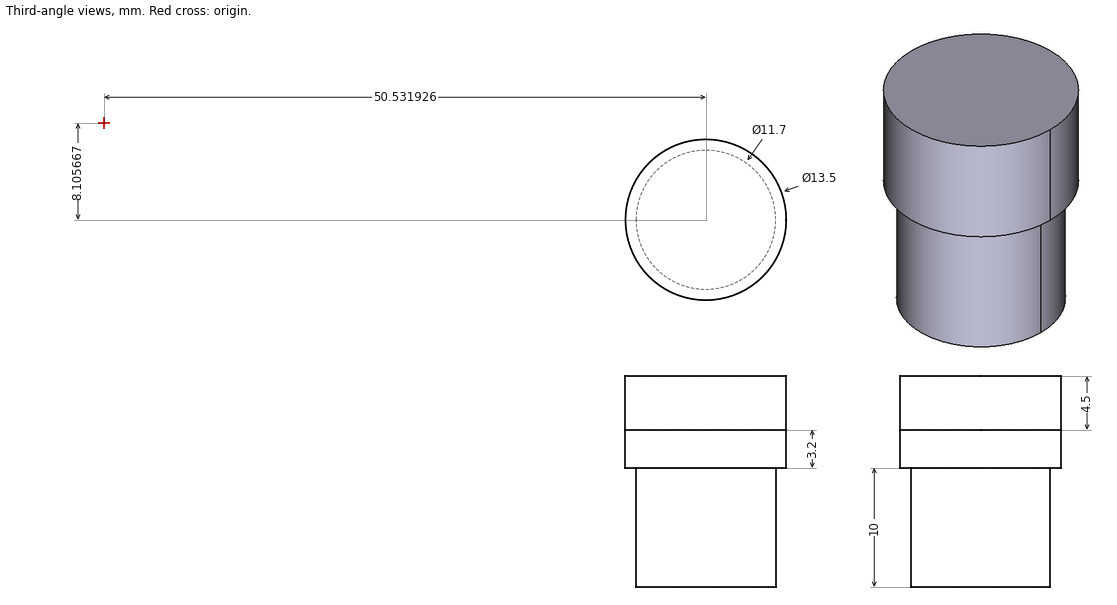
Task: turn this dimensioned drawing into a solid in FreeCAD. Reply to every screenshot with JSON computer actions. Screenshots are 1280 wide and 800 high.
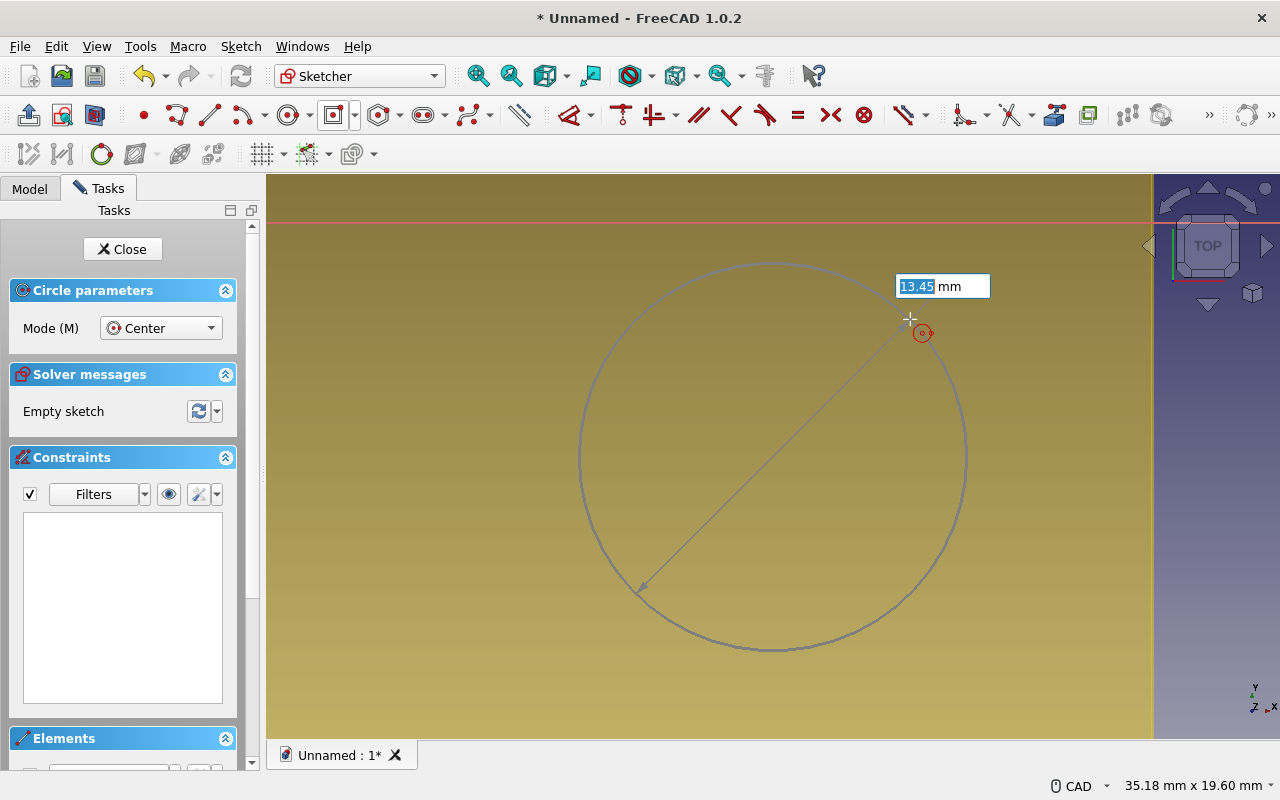
{"action": "type", "text": "13.5"}
{"action": "key", "text": "Return"}
{"action": "key", "text": "Escape"}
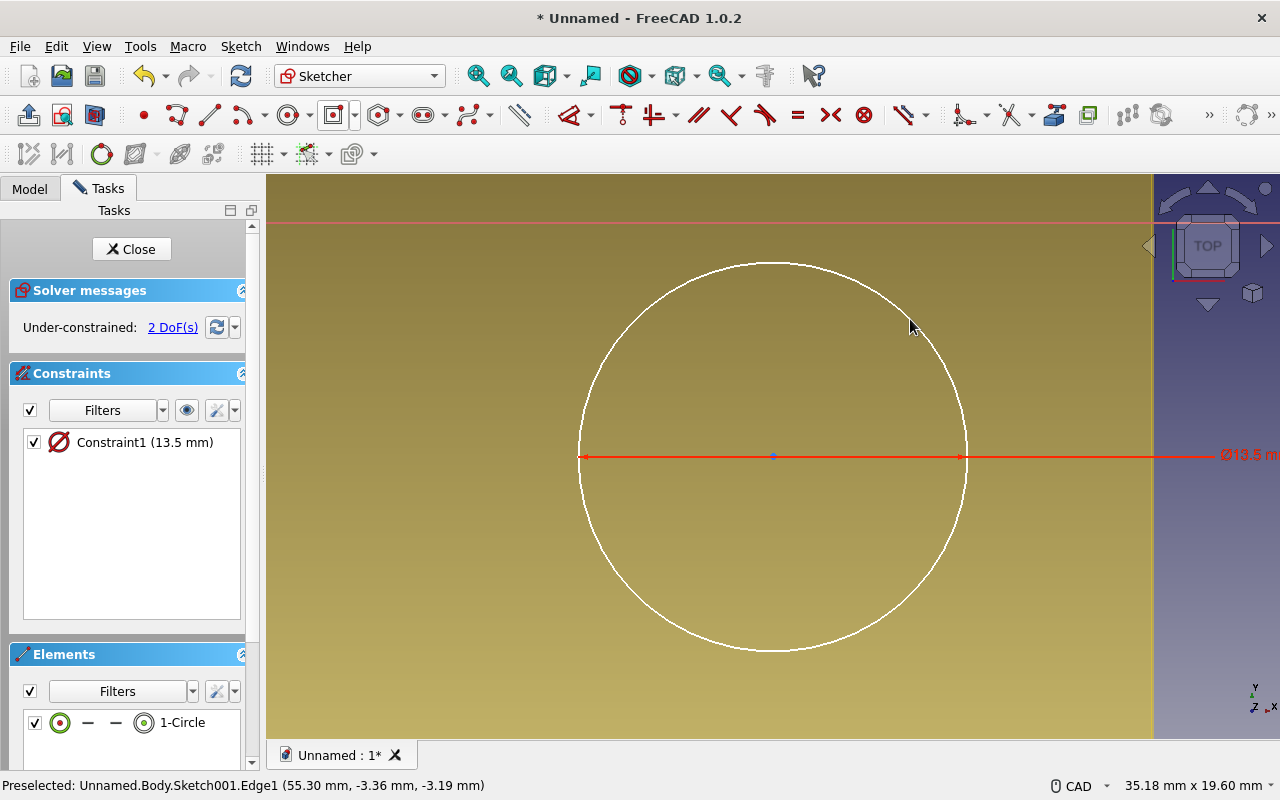
{"action": "key", "text": "d"}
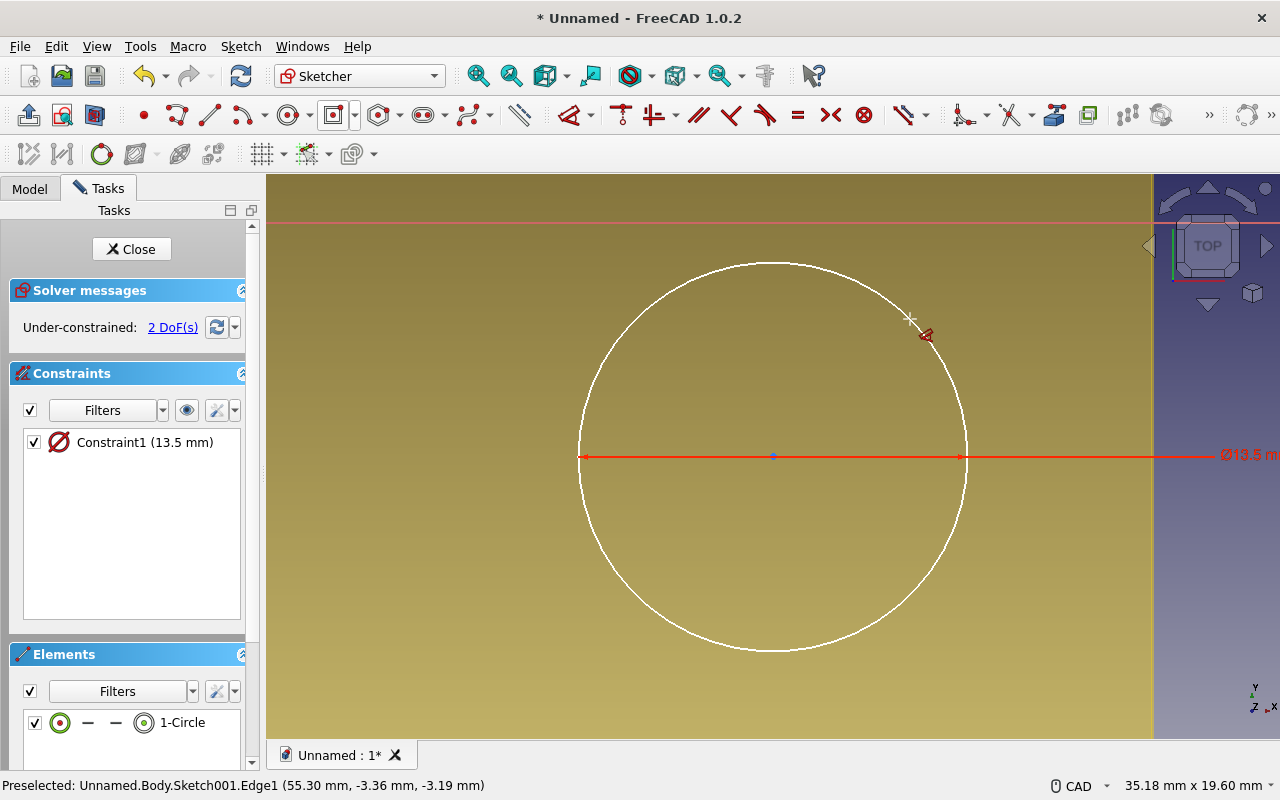
{"action": "left_click", "coordinate": [773, 457]}
{"action": "left_click", "coordinate": [807, 340]}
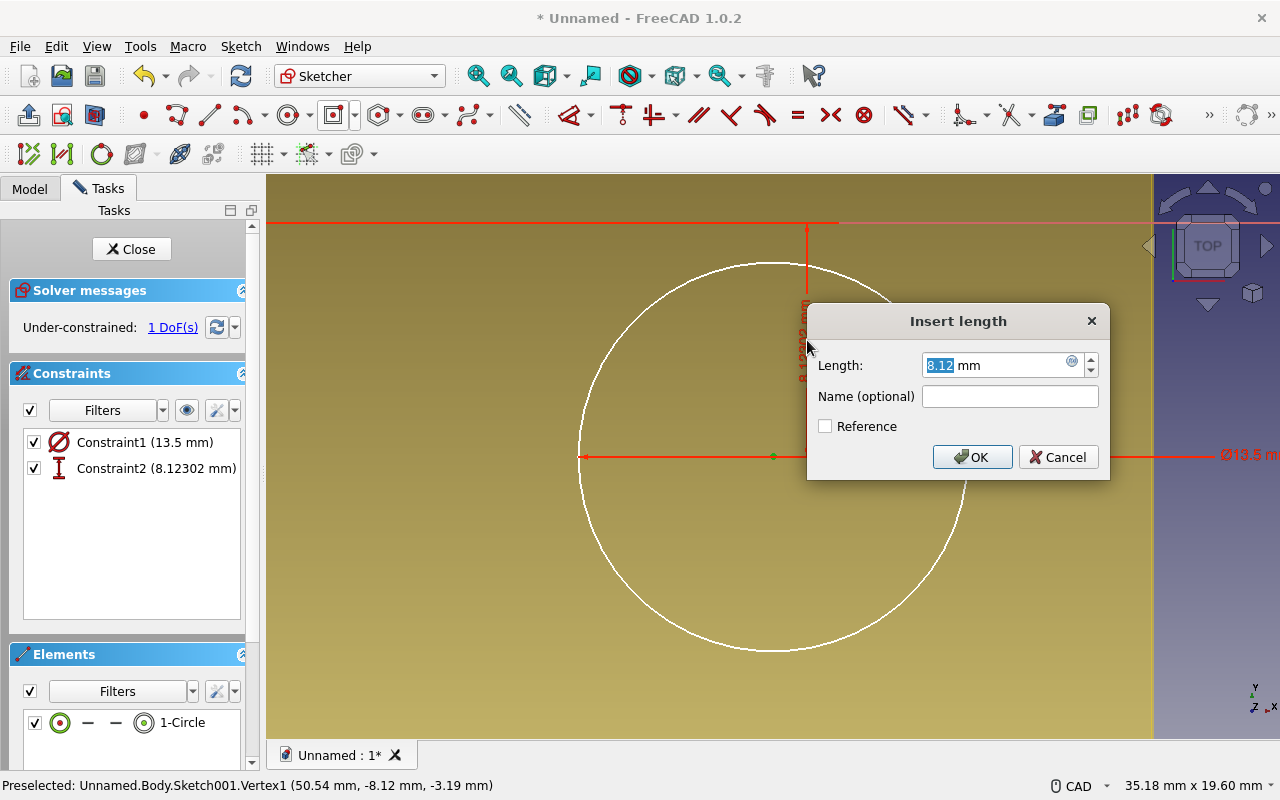
{"action": "type", "text": "8.105667"}
{"action": "key", "text": "Return"}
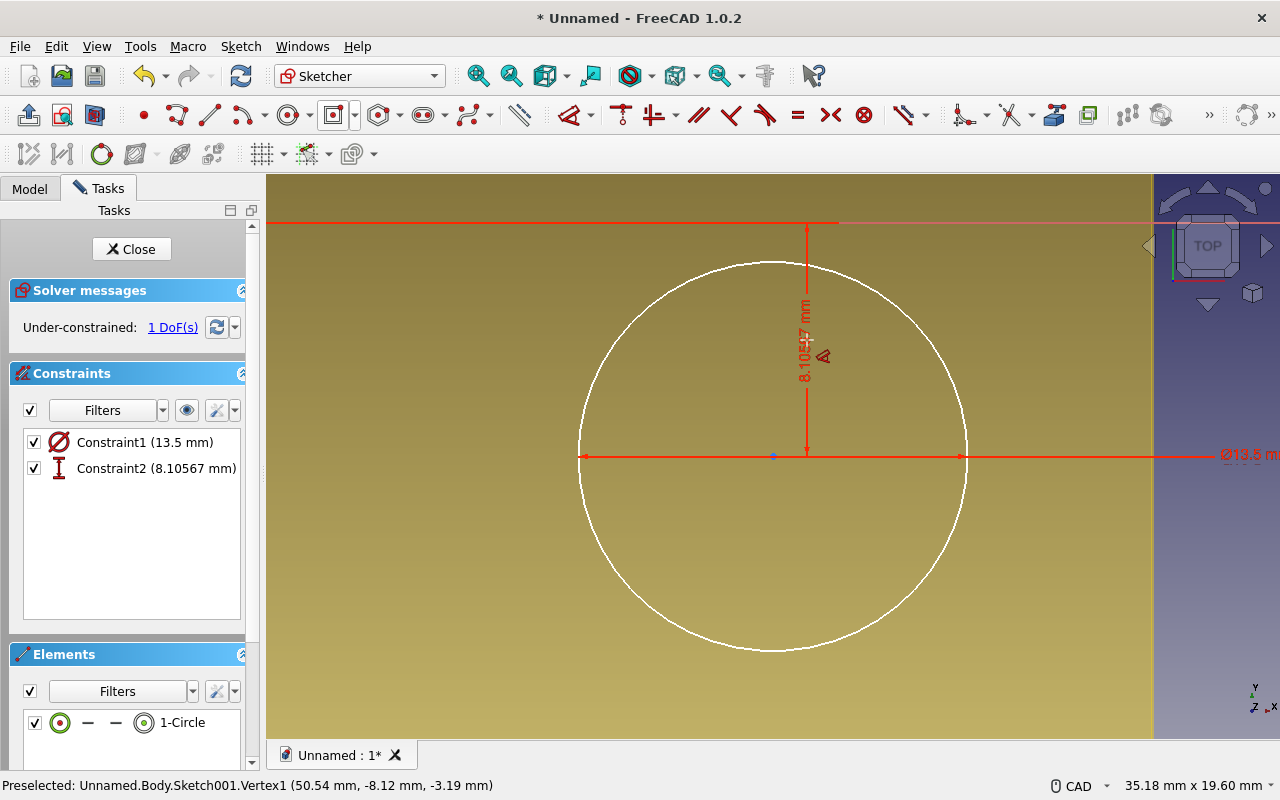
{"action": "left_click", "coordinate": [773, 456]}
{"action": "left_click", "coordinate": [533, 490]}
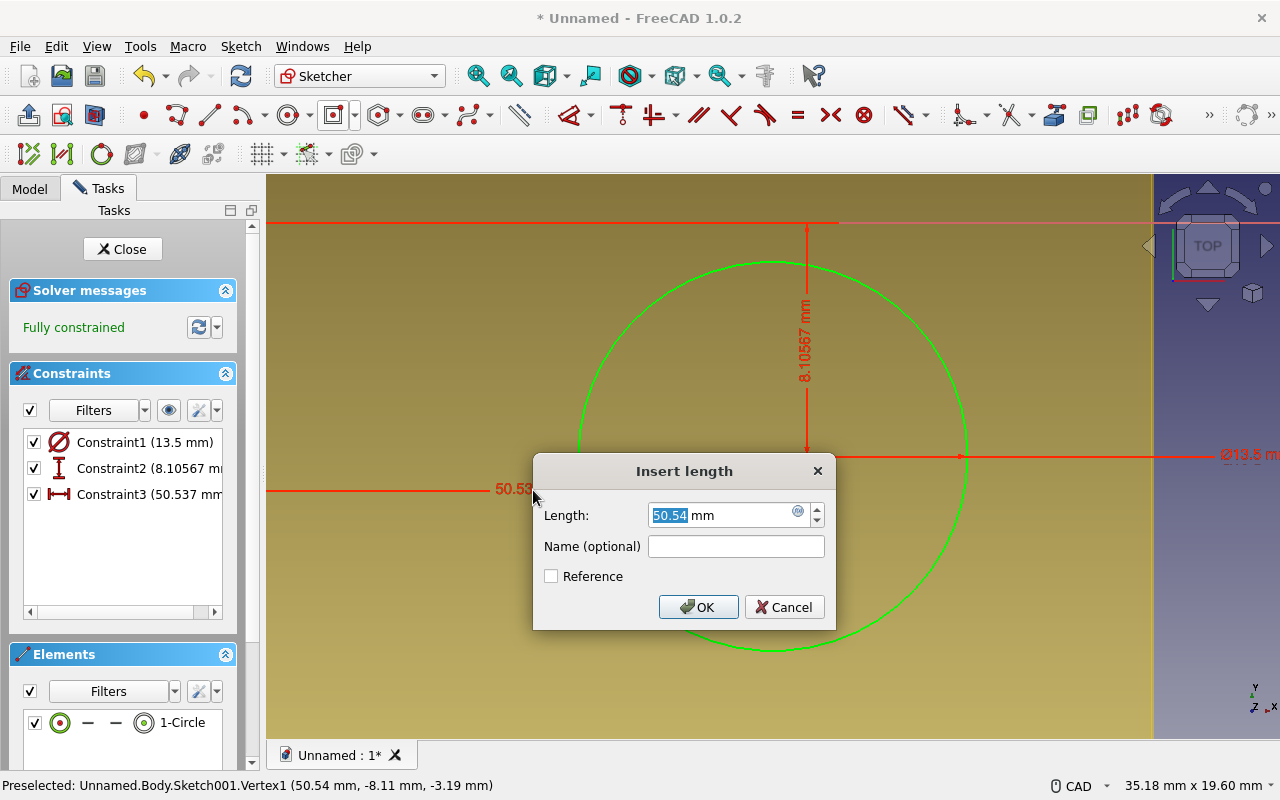
{"action": "type", "text": "50.531926"}
{"action": "key", "text": "Return"}
{"action": "key", "text": "Escape"}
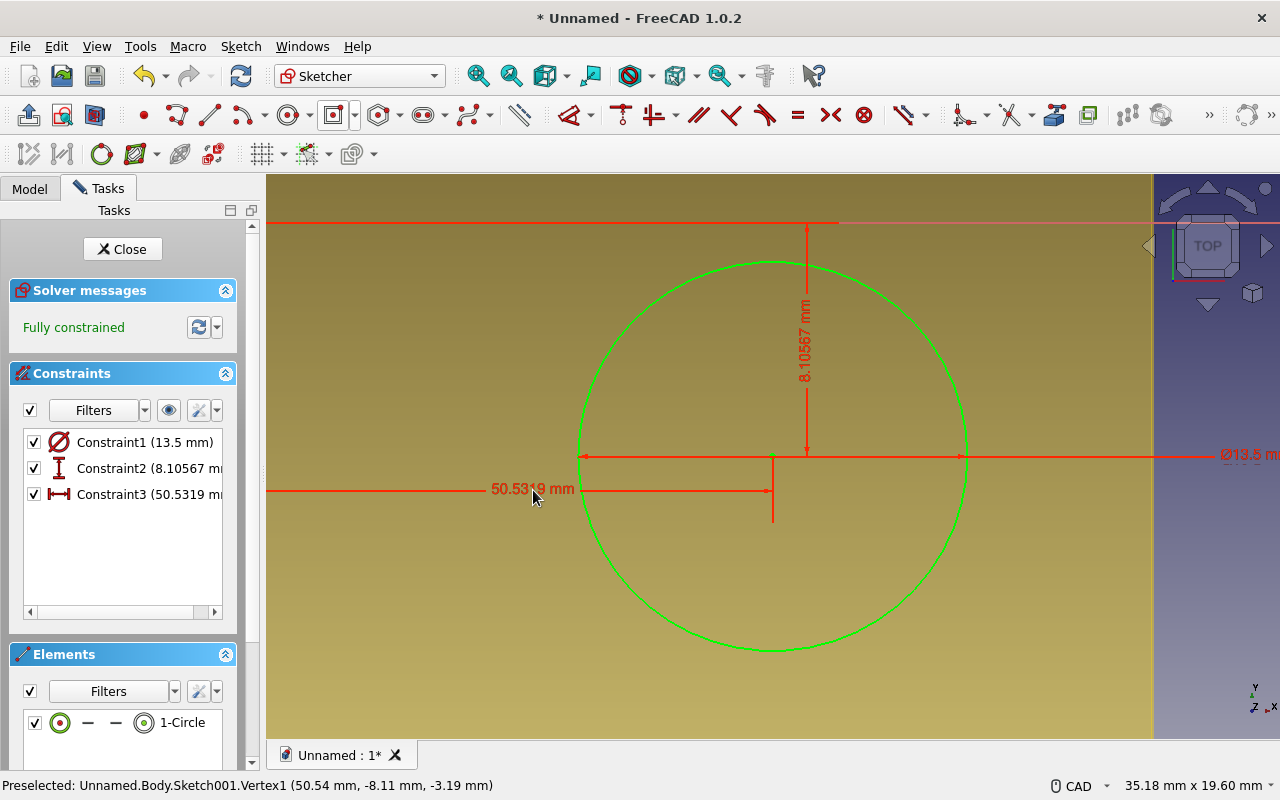
{"action": "left_click", "coordinate": [123, 249]}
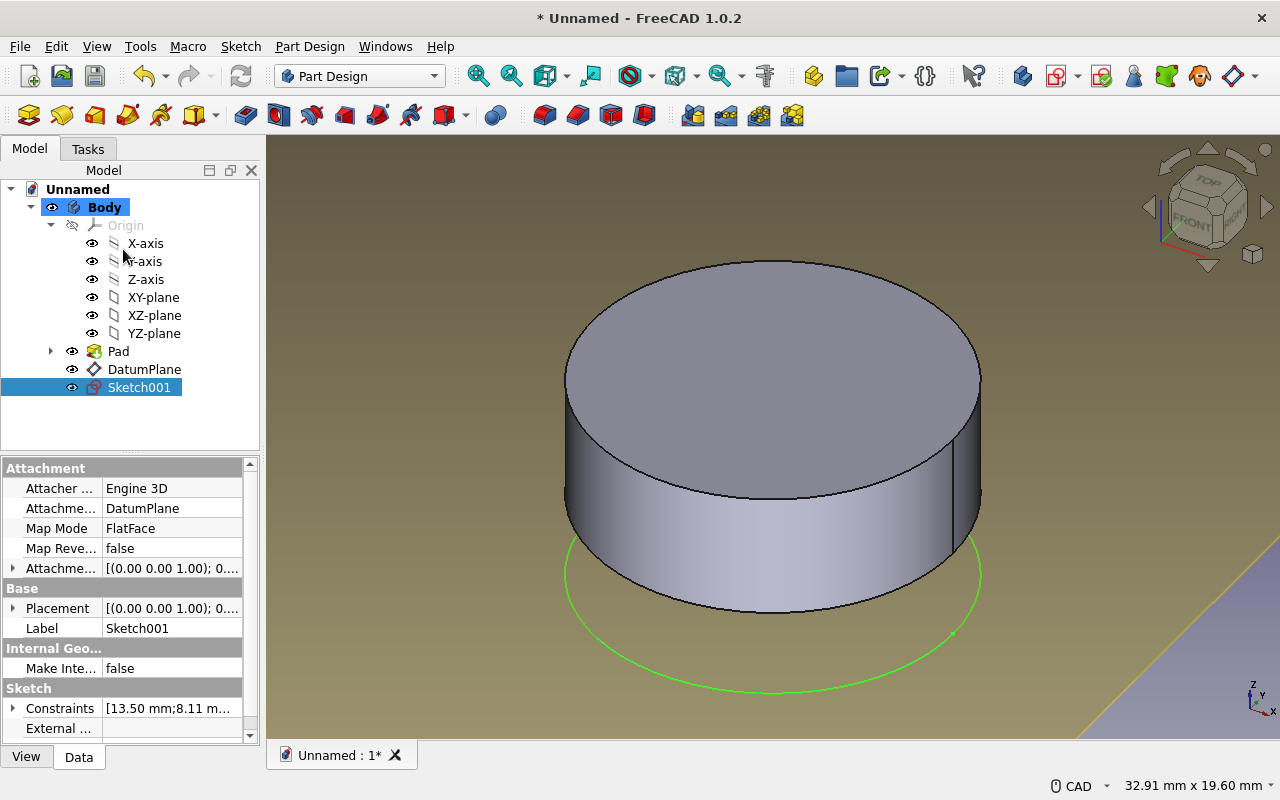
{"action": "left_click", "coordinate": [29, 116]}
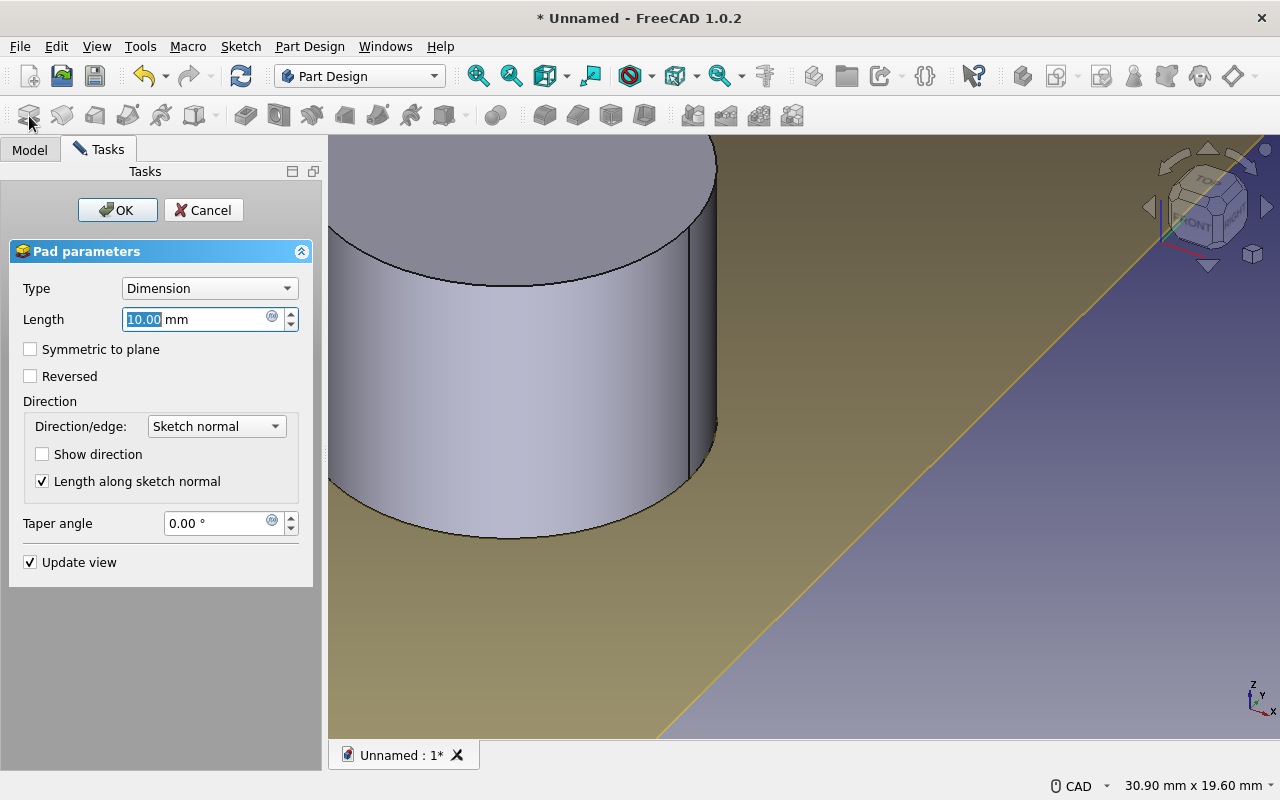
{"action": "type", "text": "3.2"}
{"action": "key", "text": "Tab"}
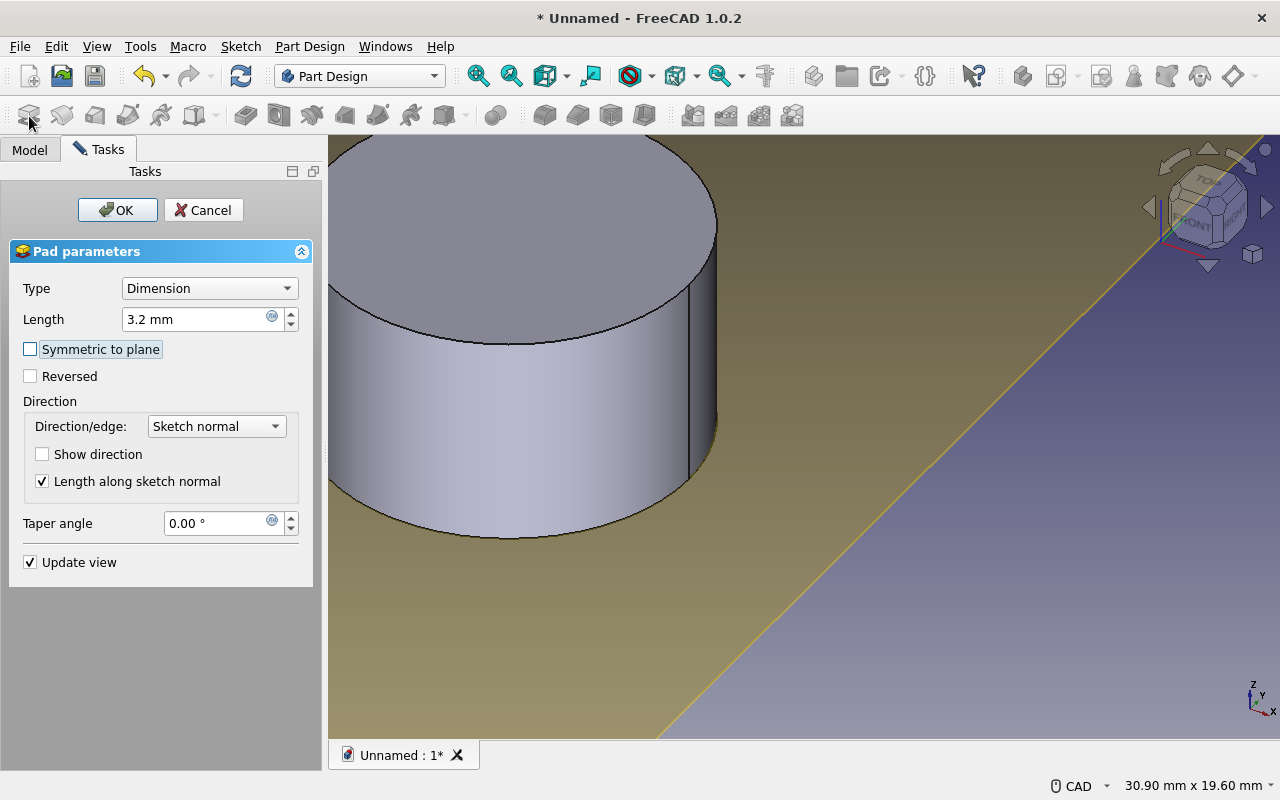
{"action": "left_click", "coordinate": [118, 210]}